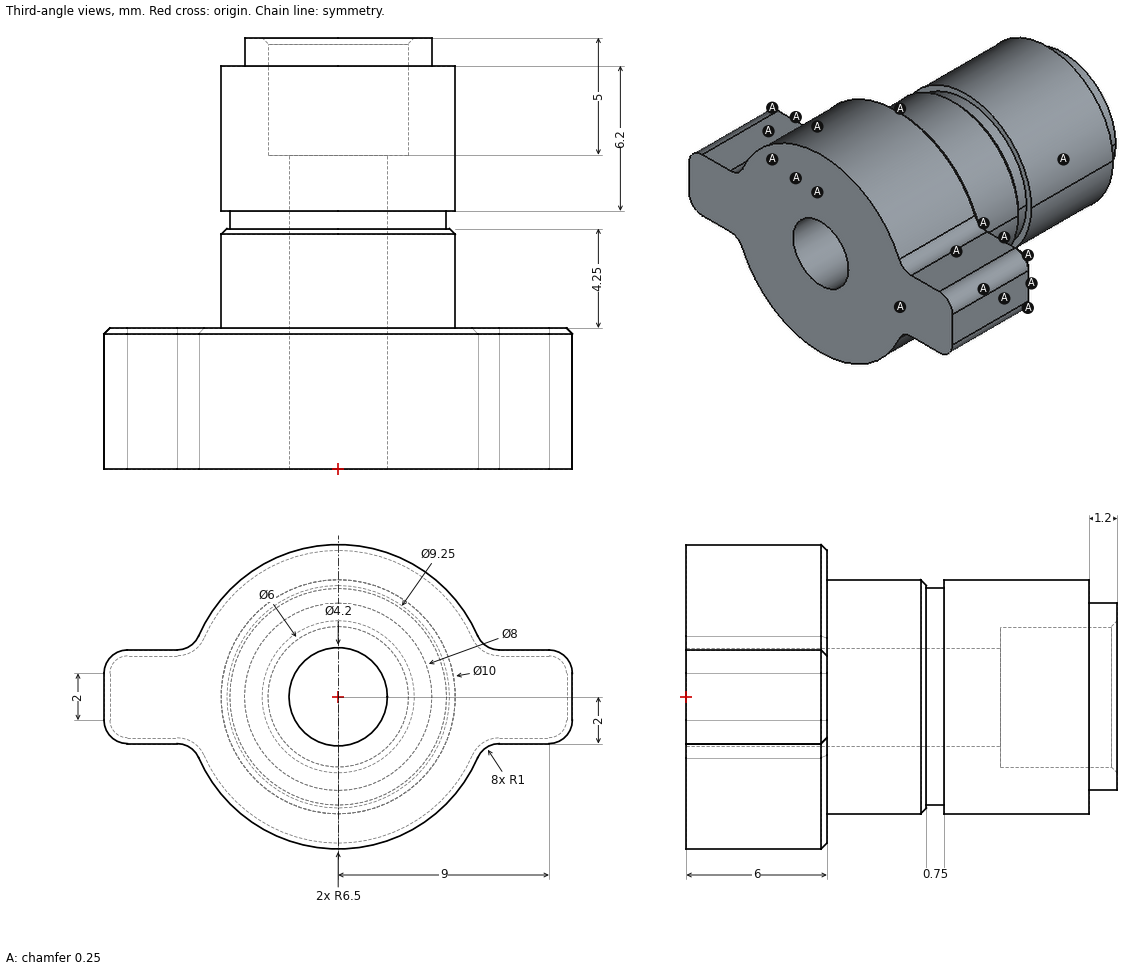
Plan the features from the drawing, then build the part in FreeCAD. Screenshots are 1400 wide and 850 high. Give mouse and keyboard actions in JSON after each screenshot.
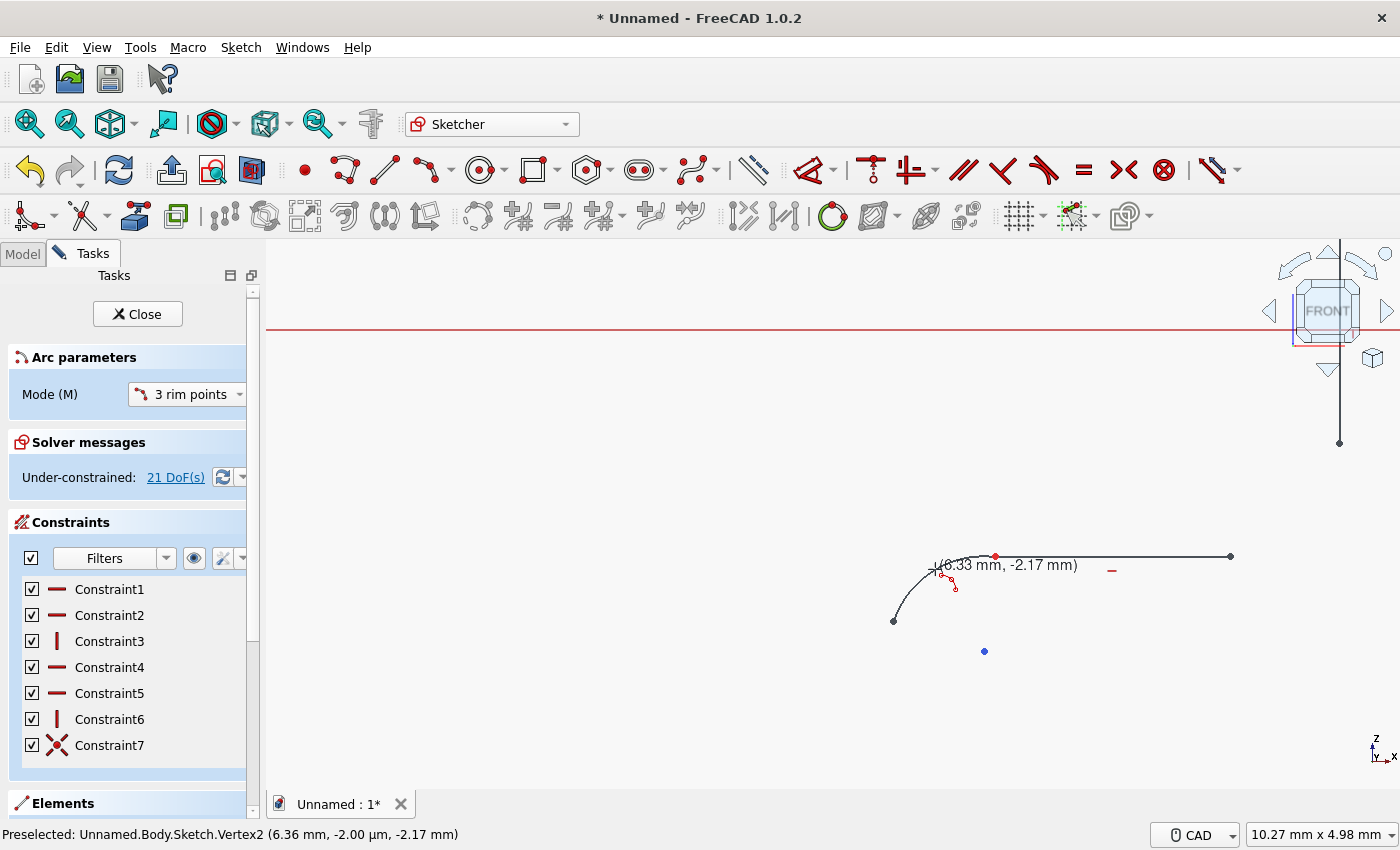
{"action": "scroll", "coordinate": [938, 574], "scroll_direction": "down", "scroll_amount": 7}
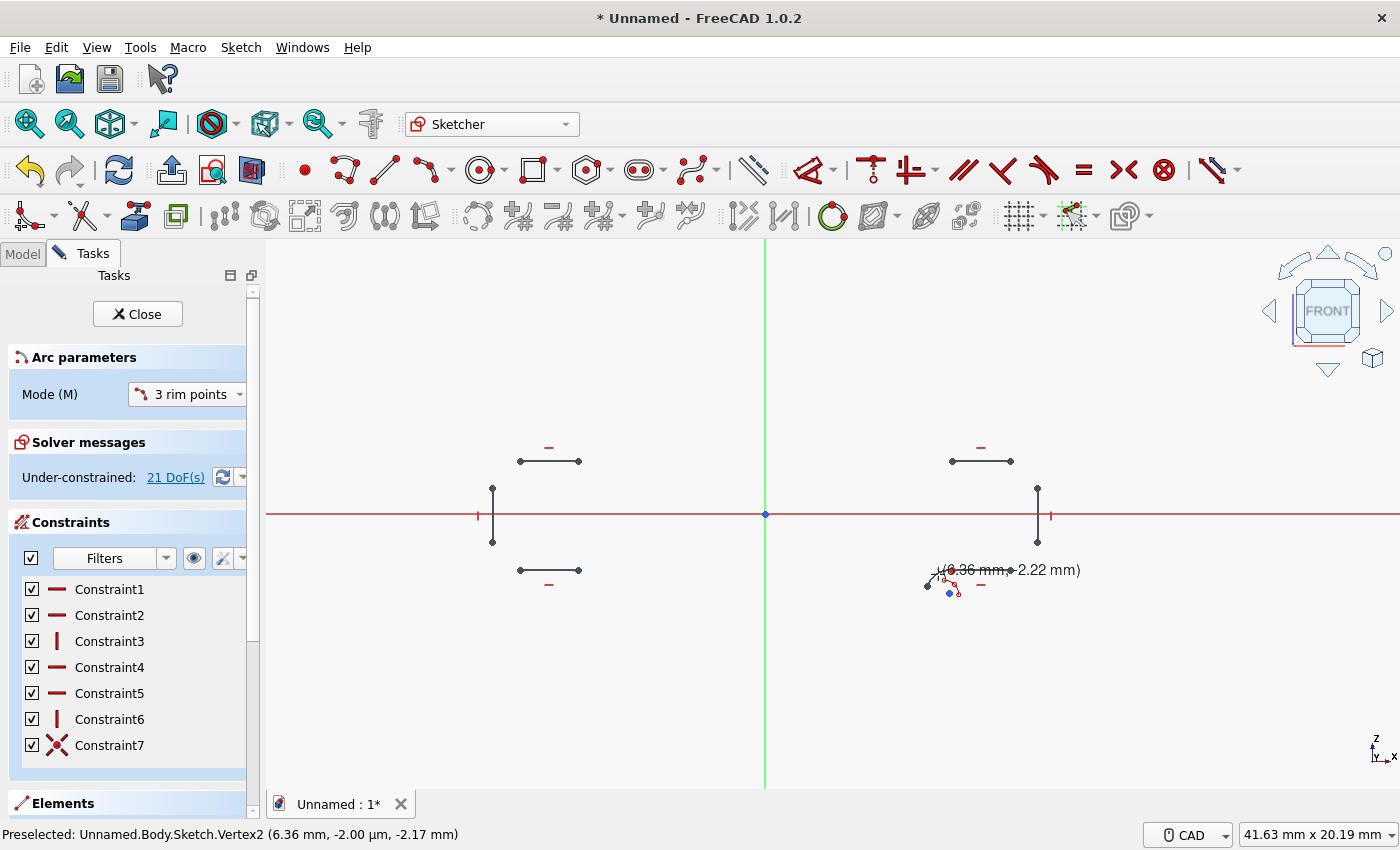
{"action": "left_click", "coordinate": [928, 586]}
{"action": "left_click", "coordinate": [603, 585]}
{"action": "left_click", "coordinate": [725, 687]}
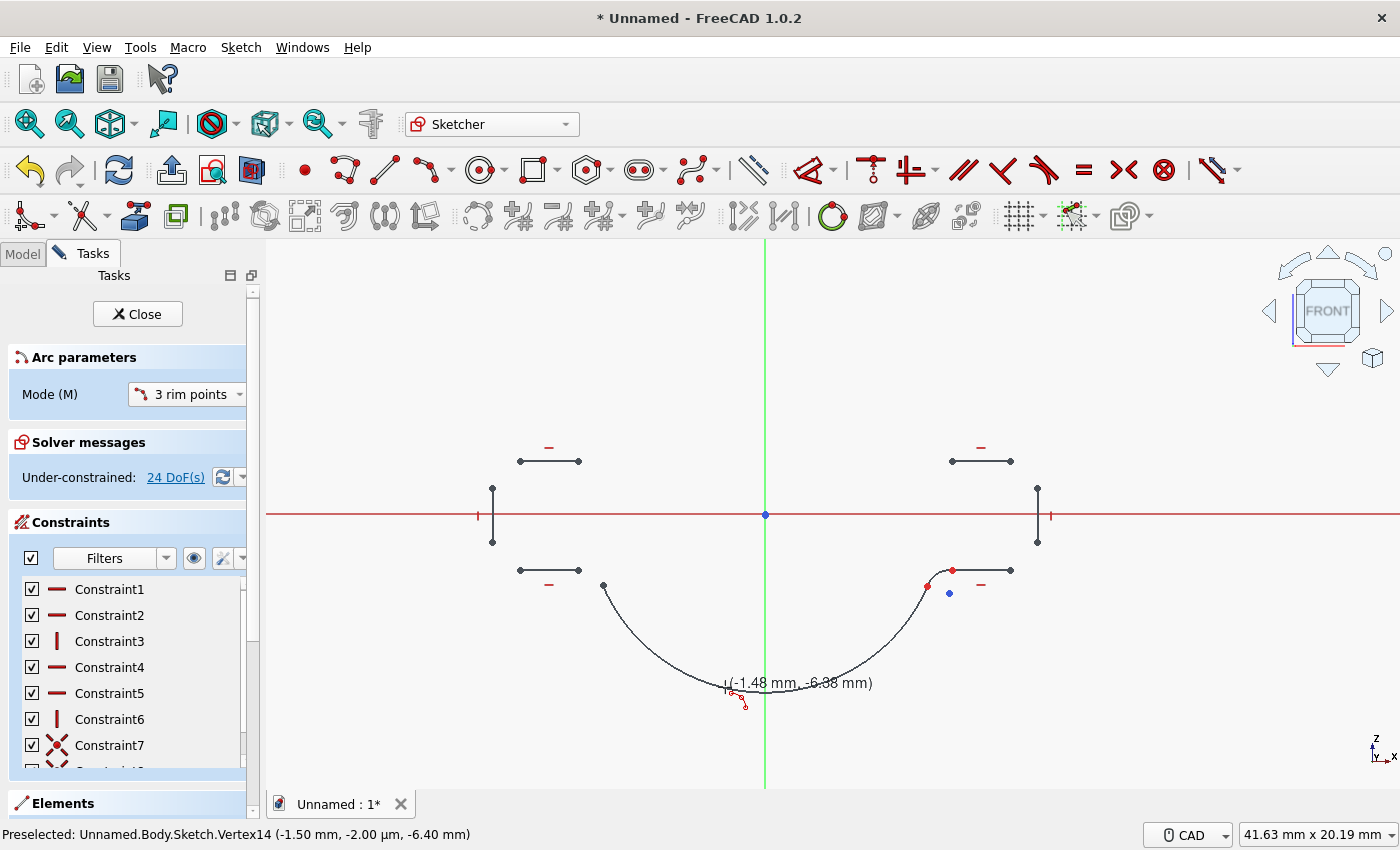
{"action": "left_click", "coordinate": [603, 586]}
{"action": "left_click", "coordinate": [579, 570]}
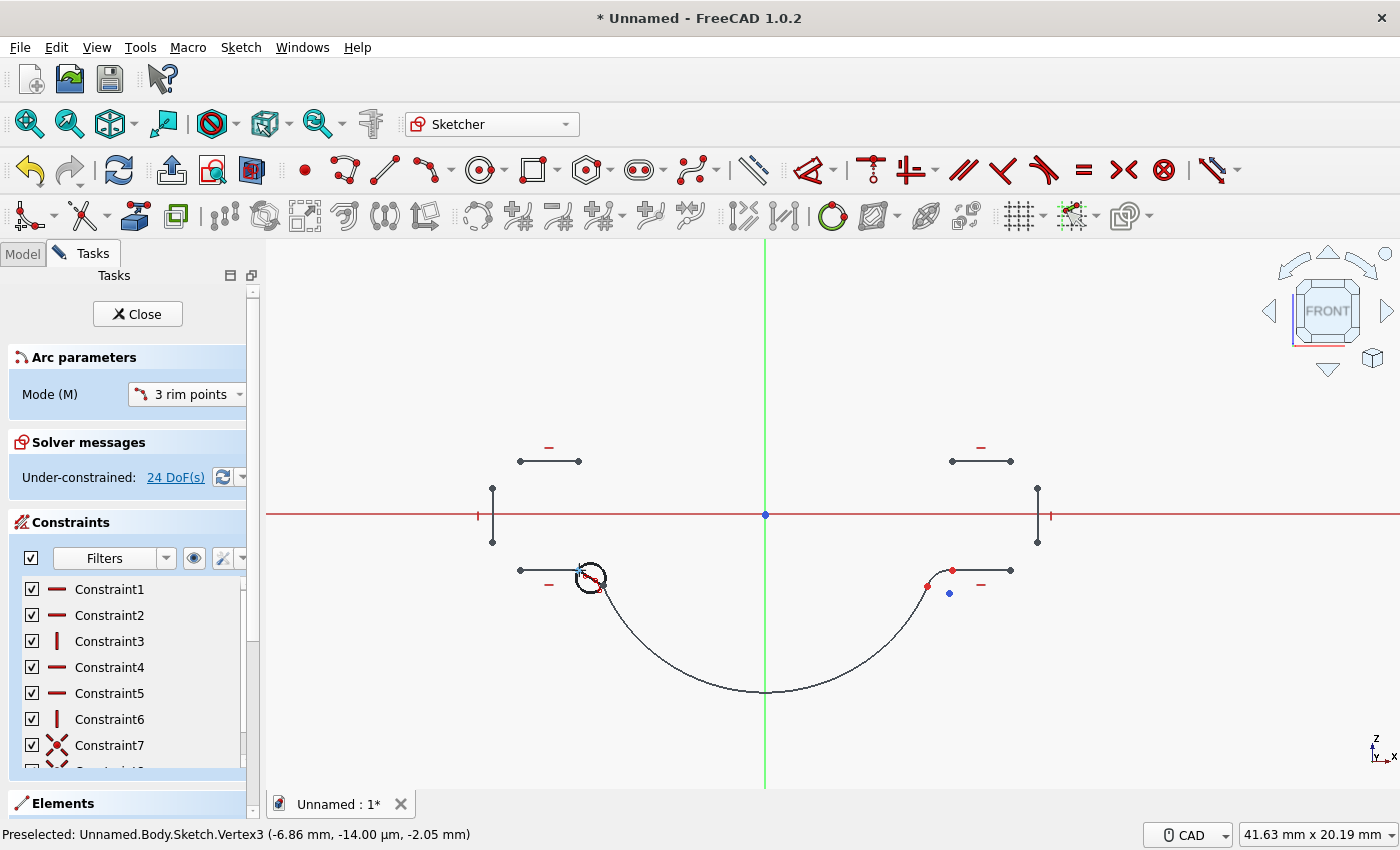
{"action": "scroll", "coordinate": [593, 573], "scroll_direction": "up", "scroll_amount": 7}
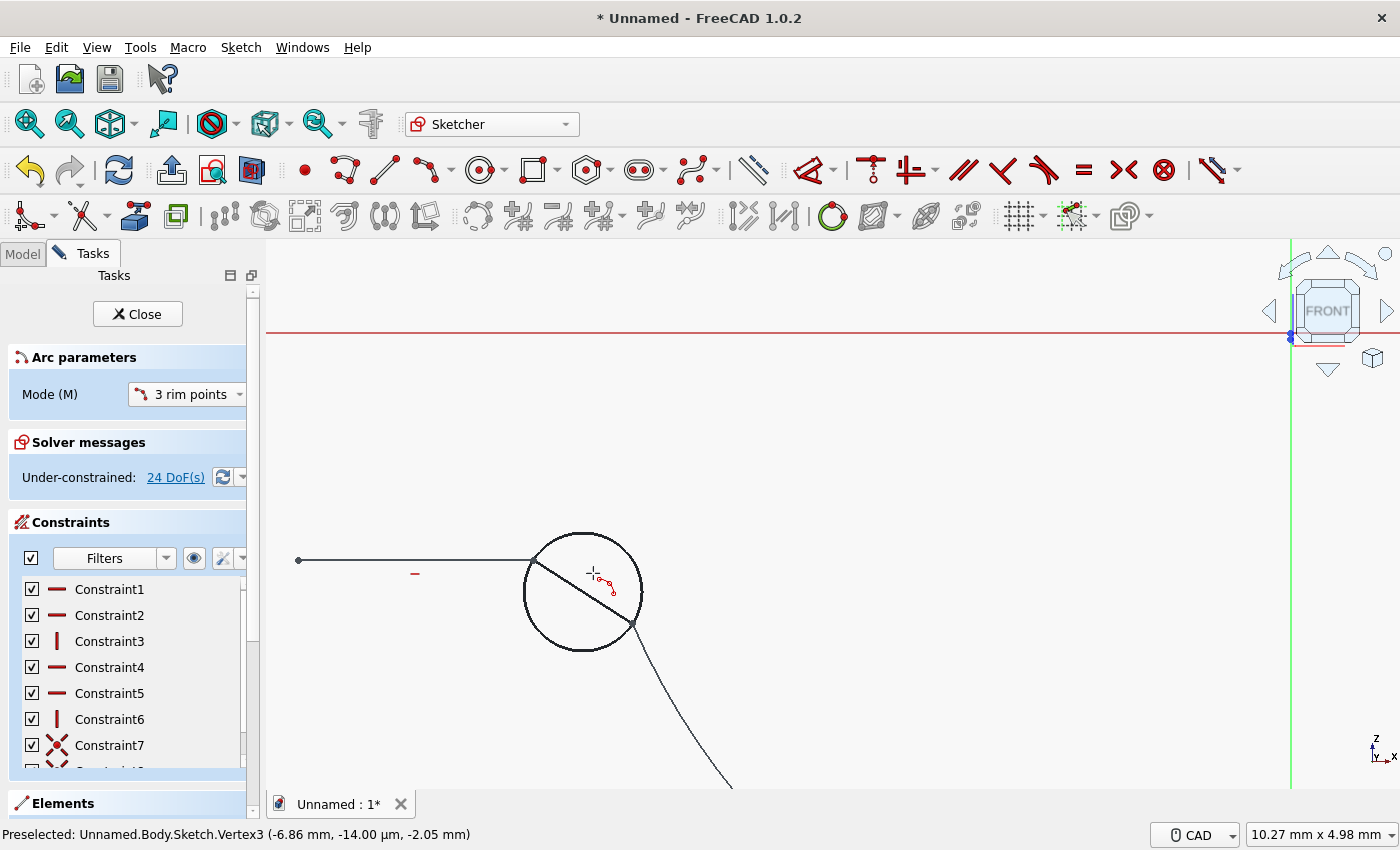
{"action": "left_click", "coordinate": [592, 572]}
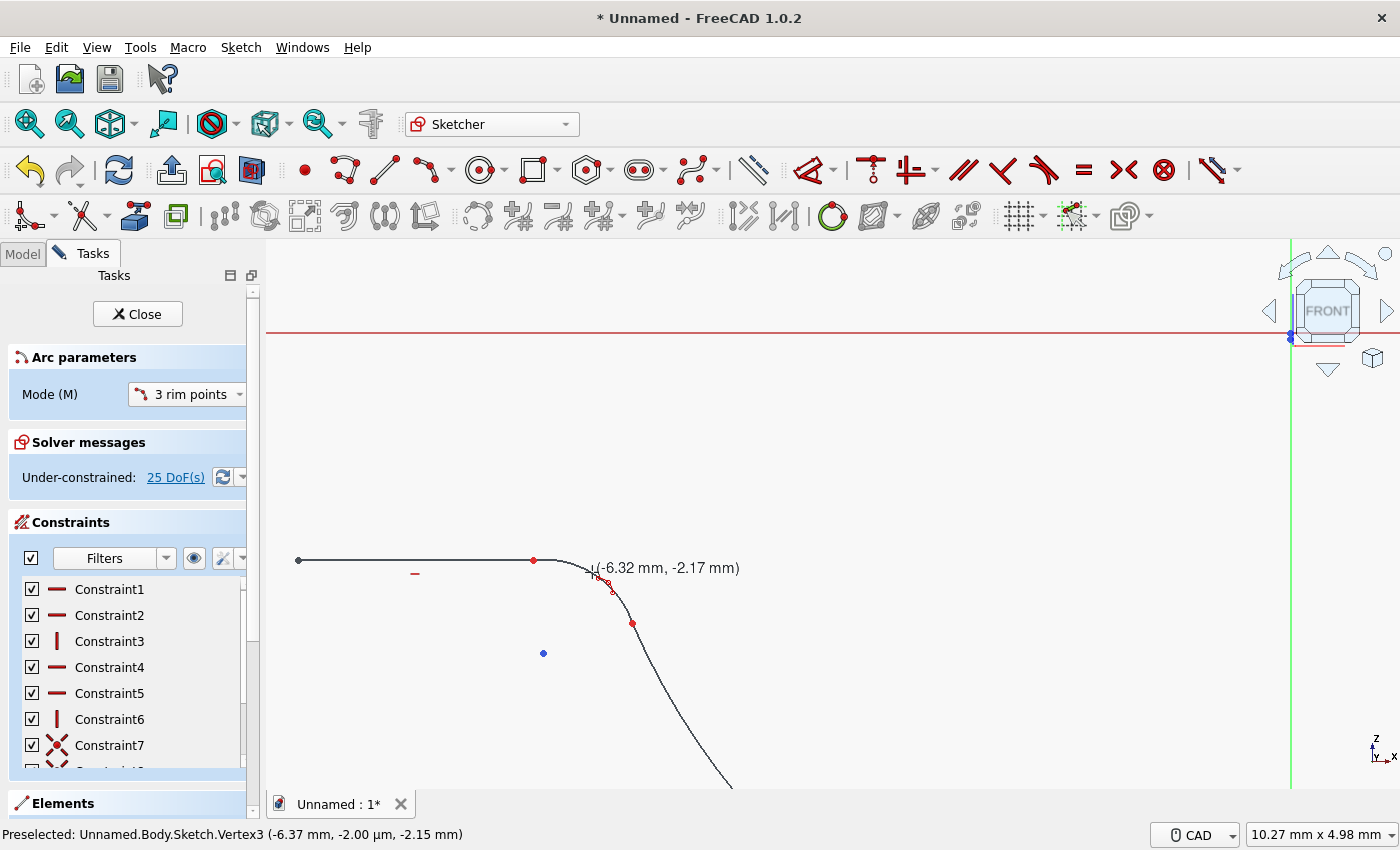
{"action": "scroll", "coordinate": [592, 573], "scroll_direction": "down", "scroll_amount": 7}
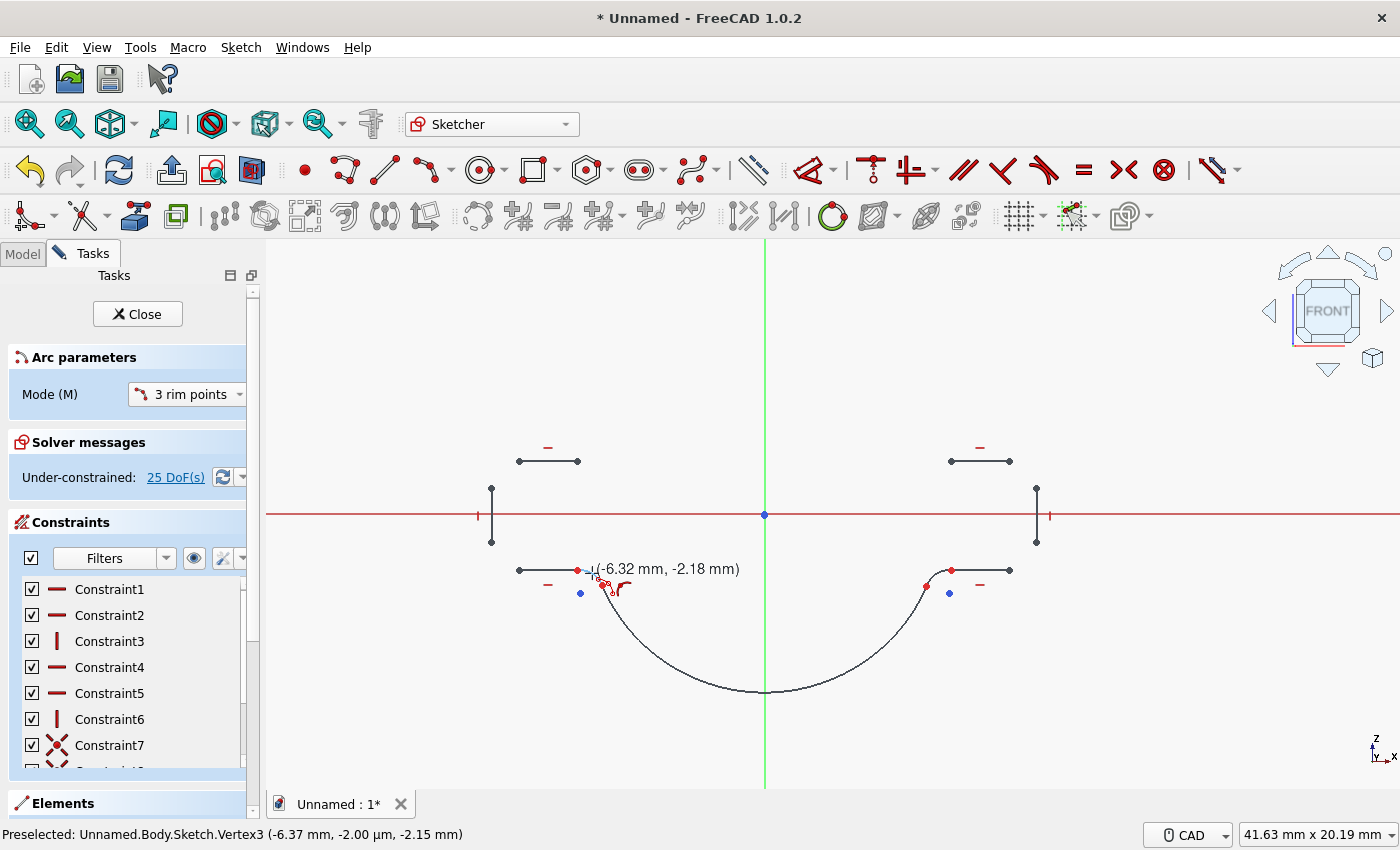
{"action": "left_click", "coordinate": [520, 570]}
{"action": "left_click", "coordinate": [492, 542]}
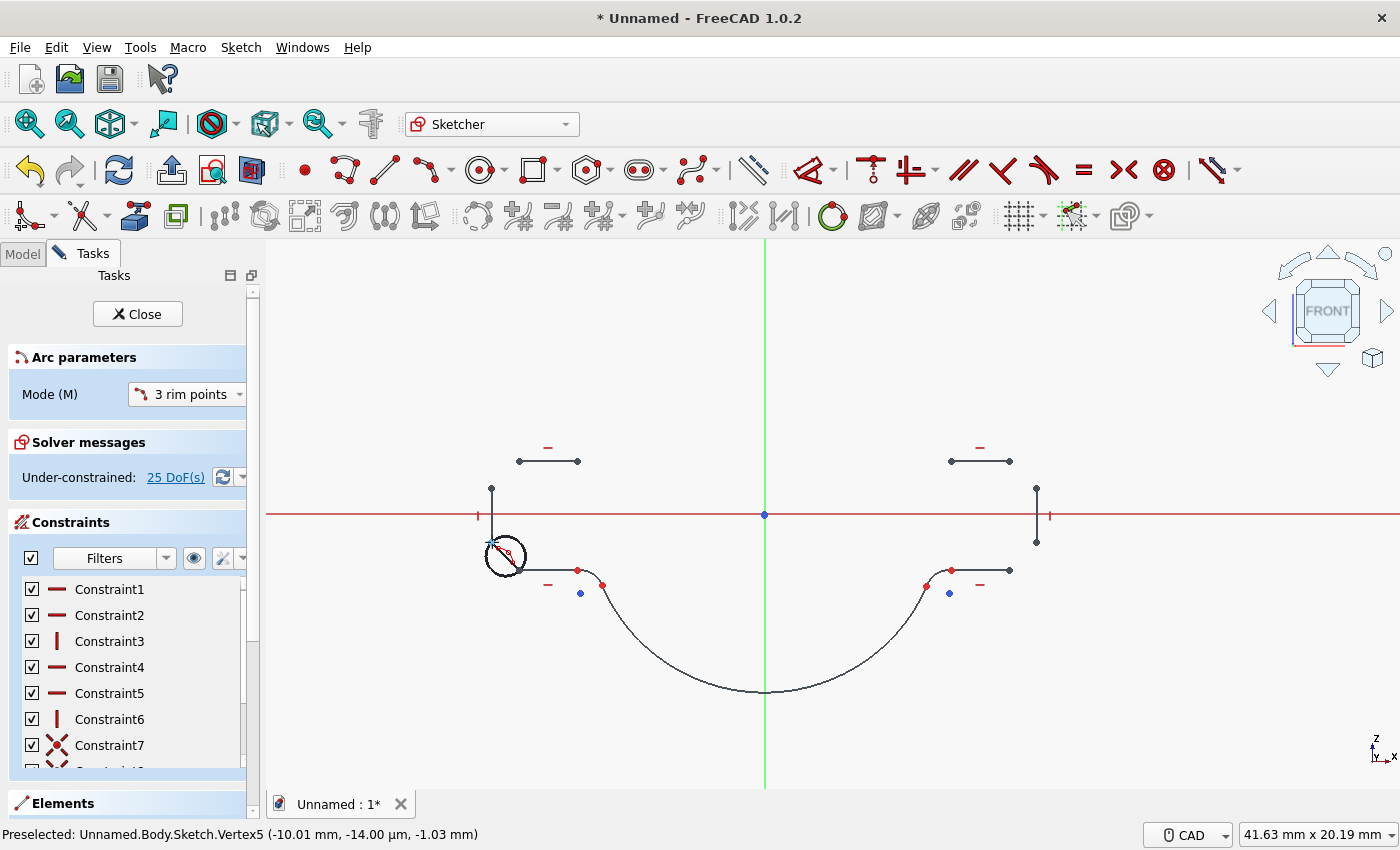
{"action": "scroll", "coordinate": [500, 561], "scroll_direction": "up", "scroll_amount": 4}